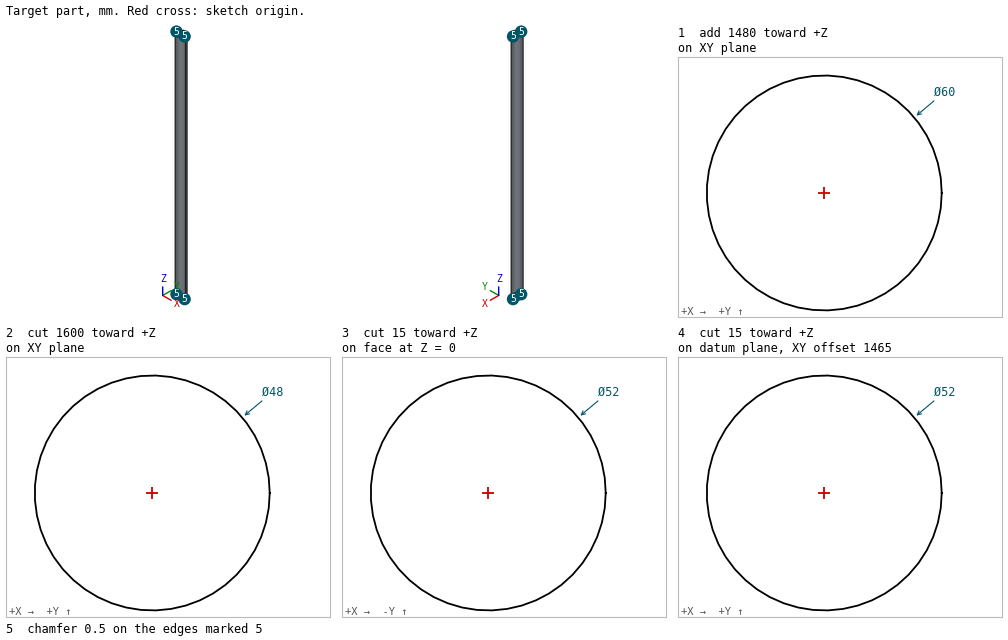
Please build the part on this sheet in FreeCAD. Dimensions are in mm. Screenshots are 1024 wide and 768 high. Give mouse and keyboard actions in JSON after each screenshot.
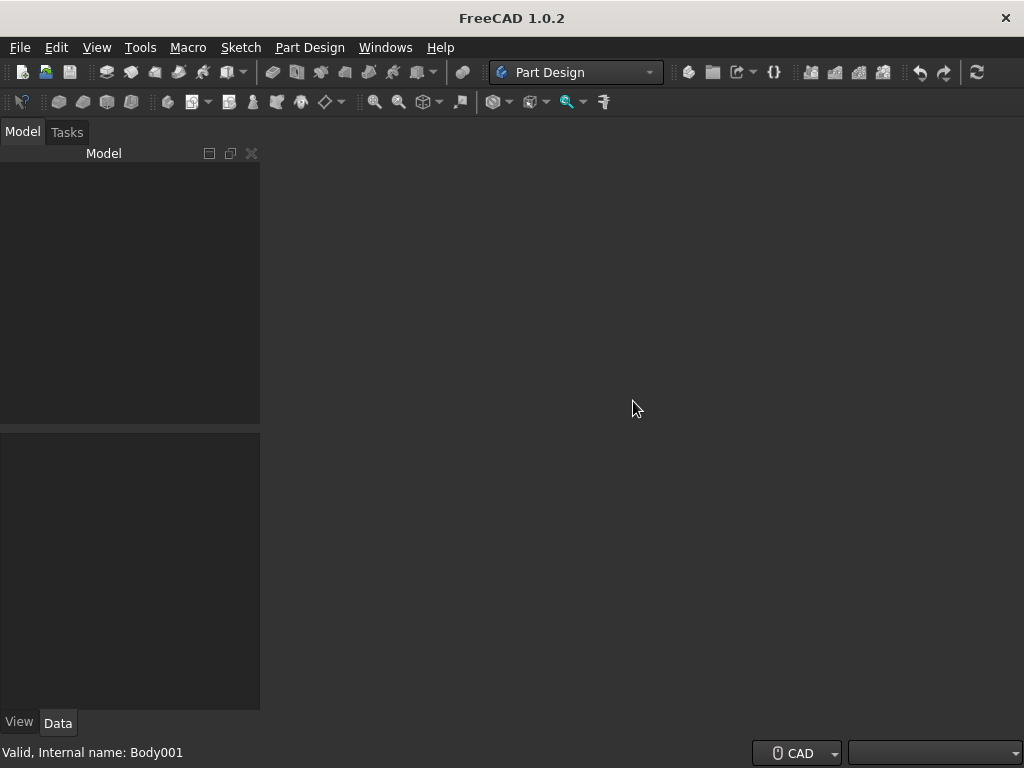
{"action": "left_click", "coordinate": [22, 72]}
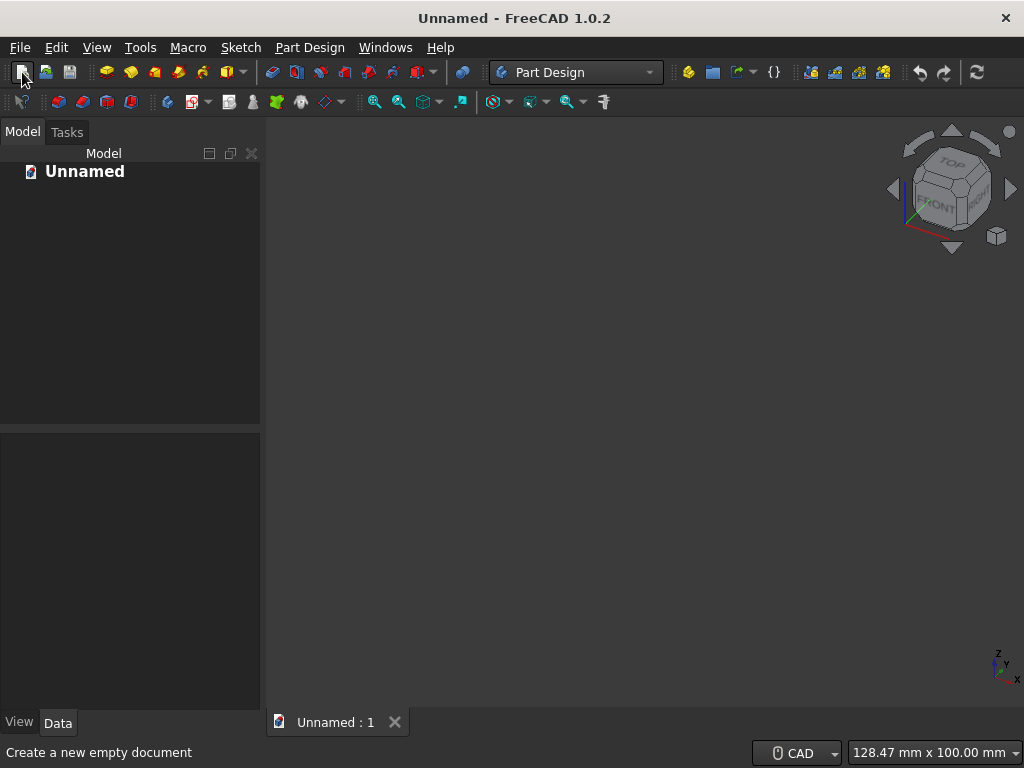
{"action": "left_click", "coordinate": [192, 102]}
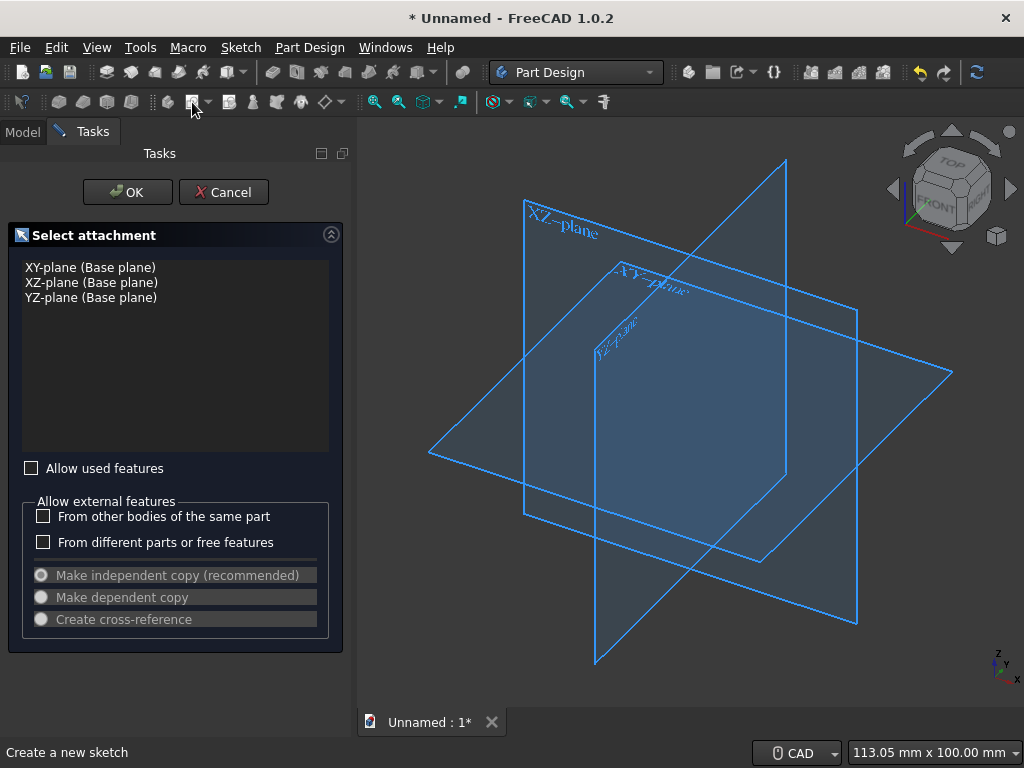
{"action": "left_click", "coordinate": [82, 268]}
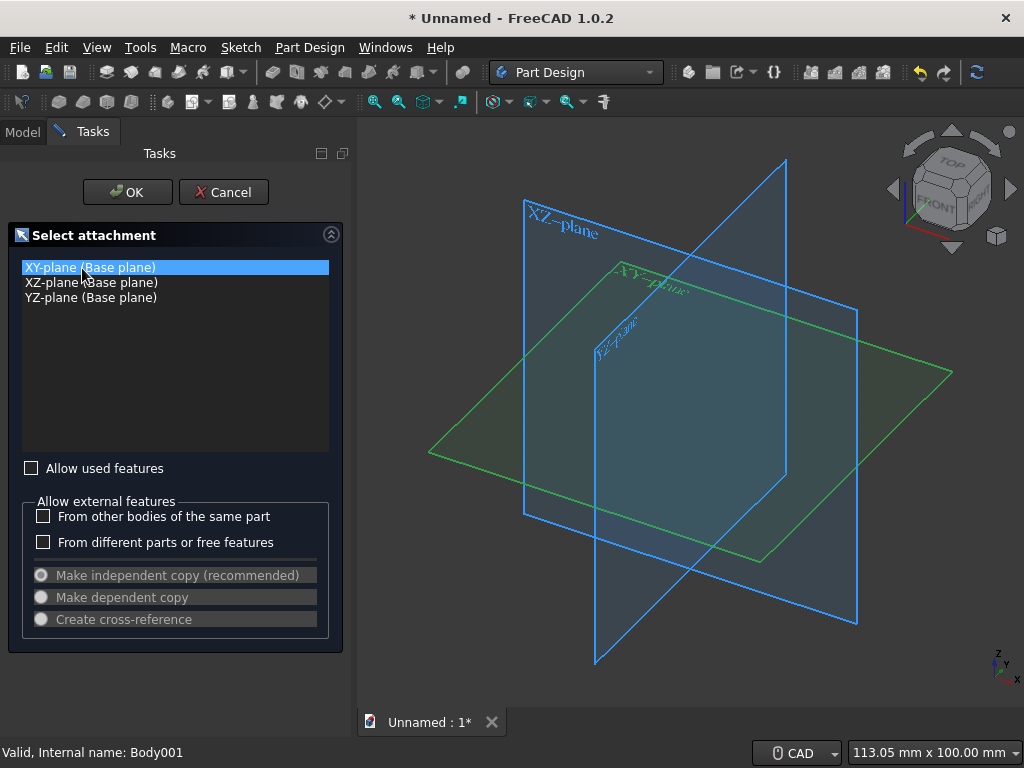
{"action": "left_click", "coordinate": [128, 192]}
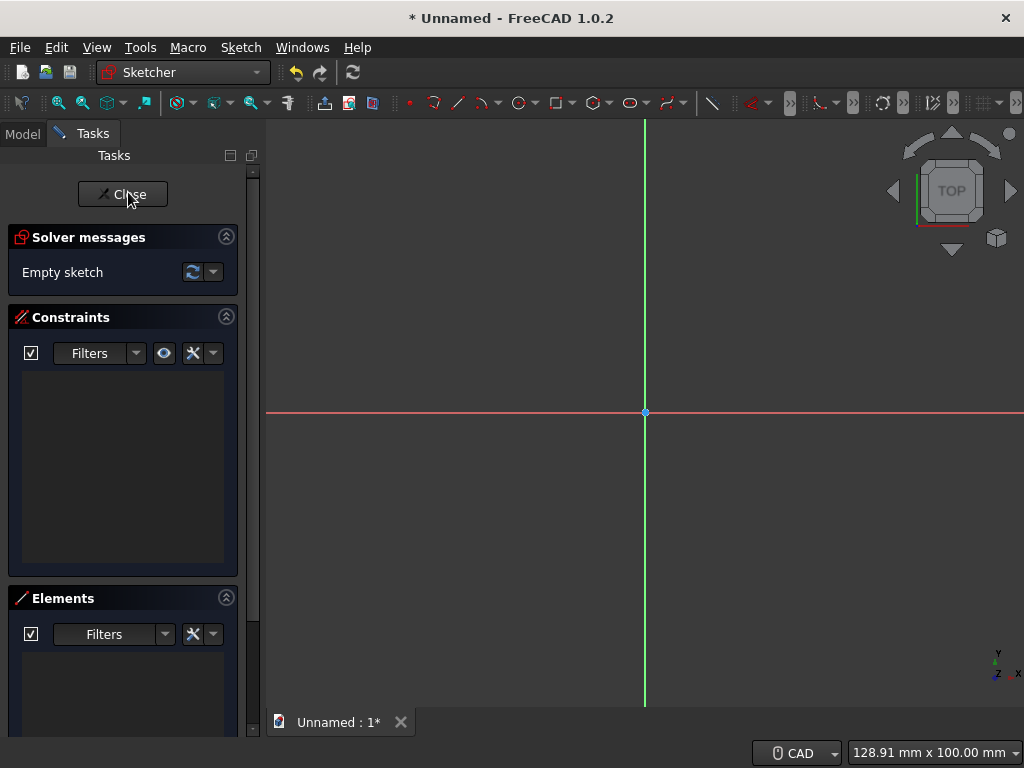
{"action": "left_click", "coordinate": [520, 104]}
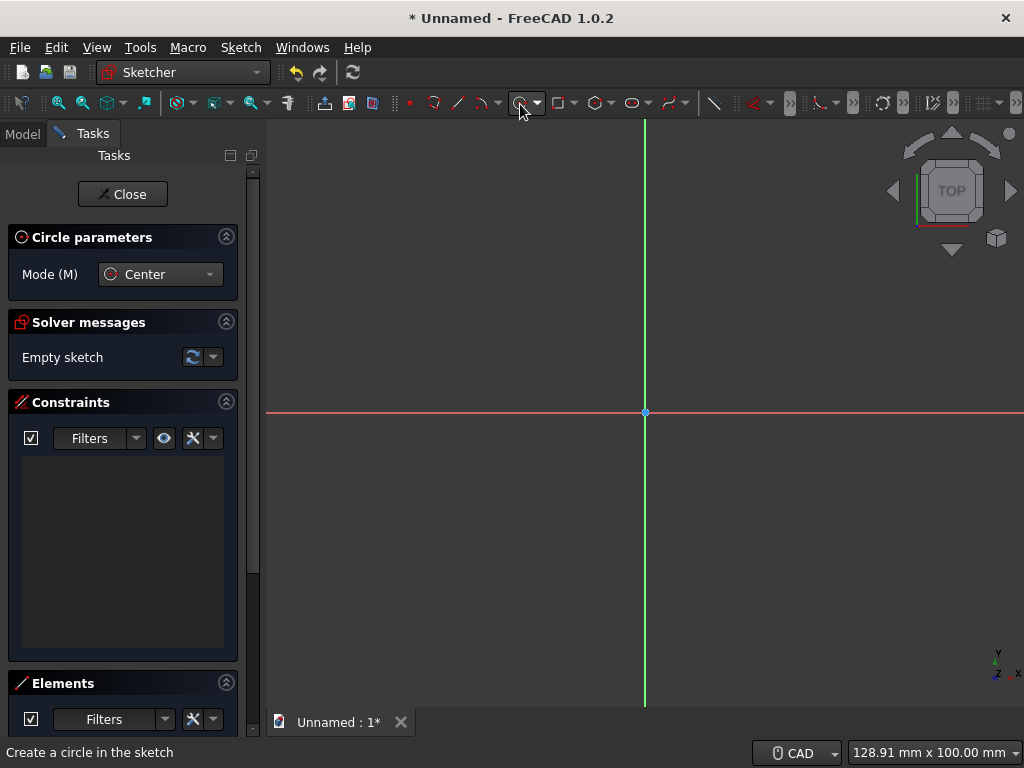
{"action": "left_click", "coordinate": [645, 413]}
{"action": "mouse_move", "coordinate": [770, 288]}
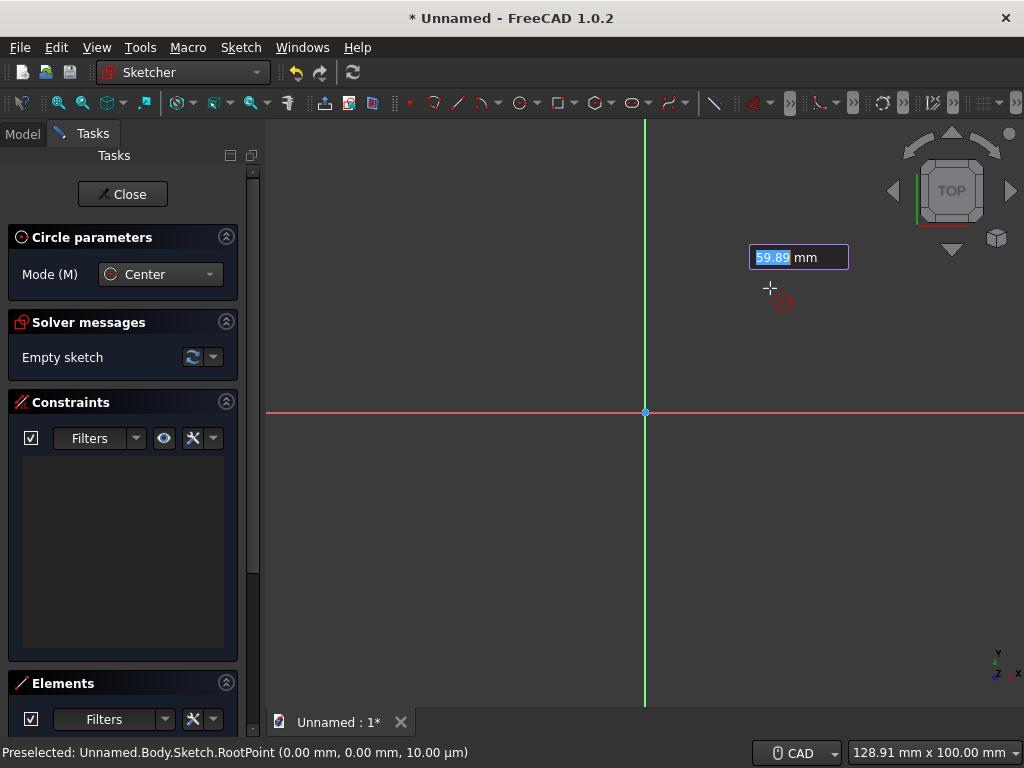
{"action": "type", "text": "60"}
{"action": "key", "text": "Return"}
{"action": "key", "text": "Escape"}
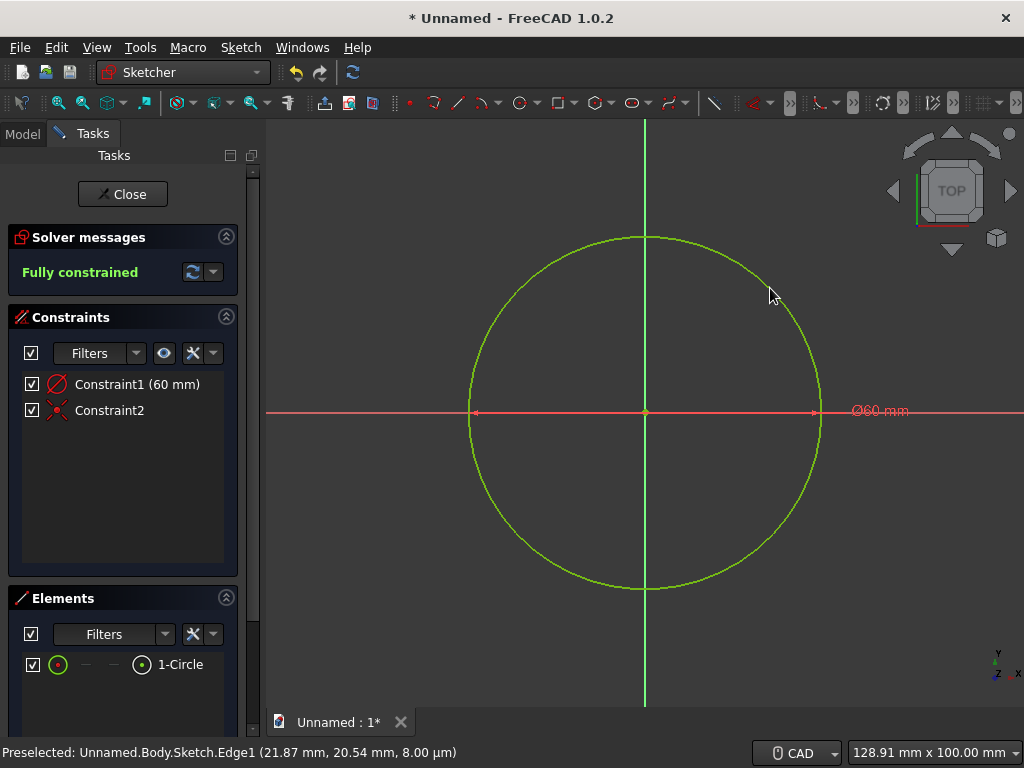
{"action": "left_click", "coordinate": [123, 194]}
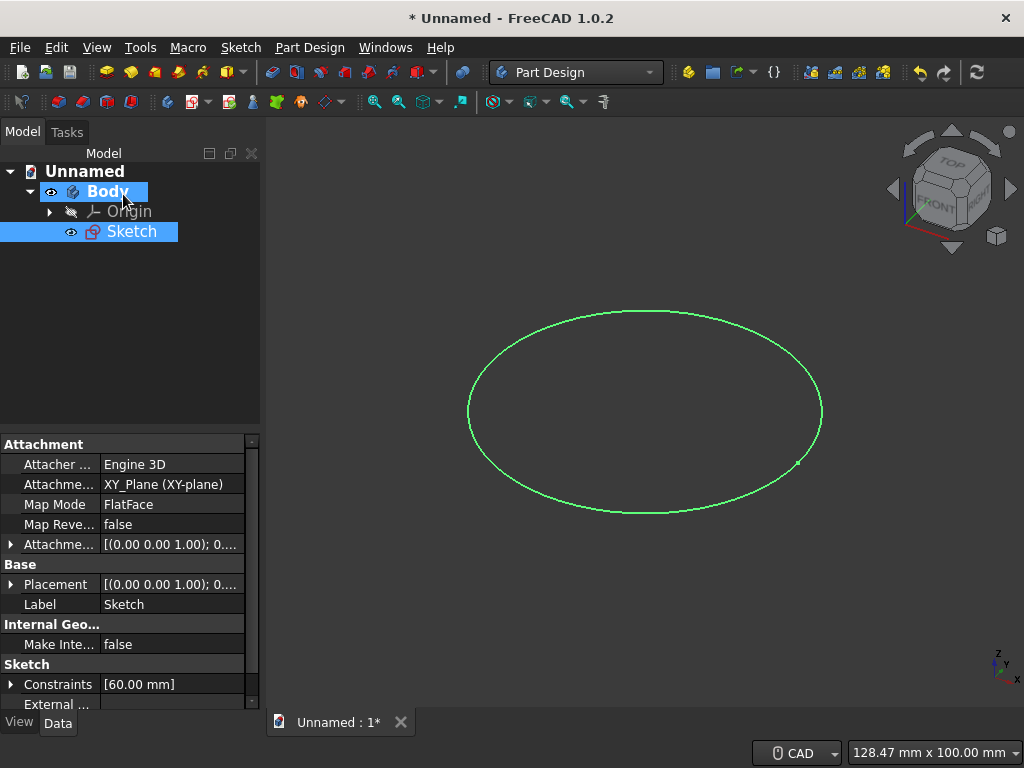
{"action": "left_click", "coordinate": [108, 72]}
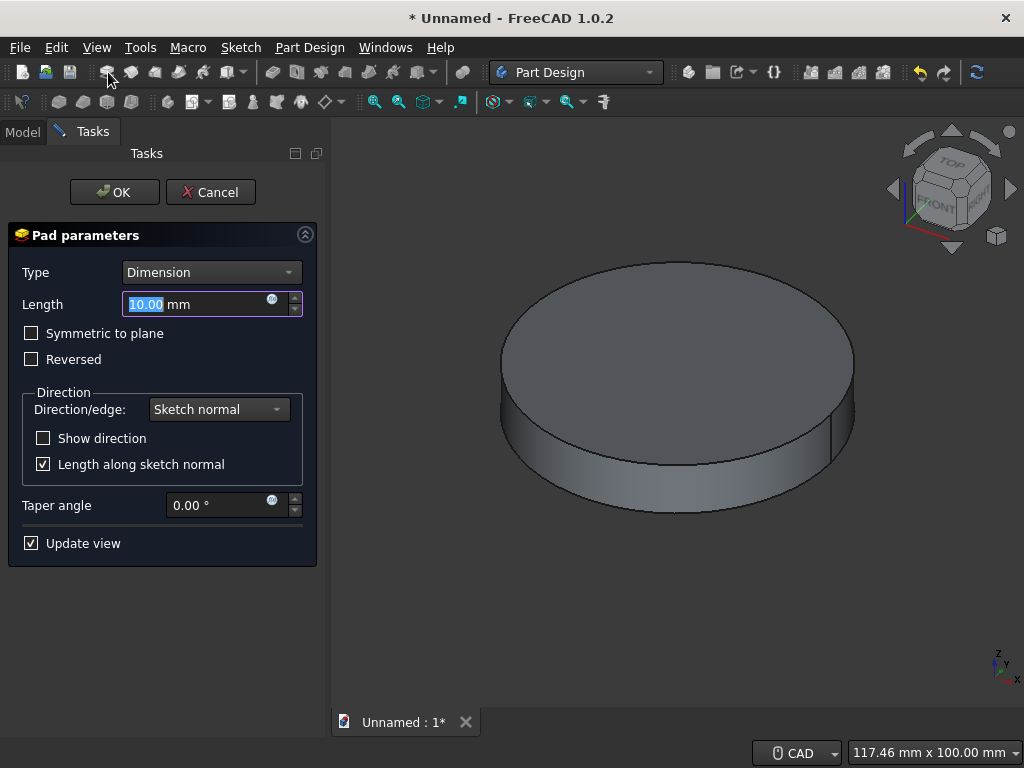
{"action": "type", "text": "1480"}
{"action": "key", "text": "Tab"}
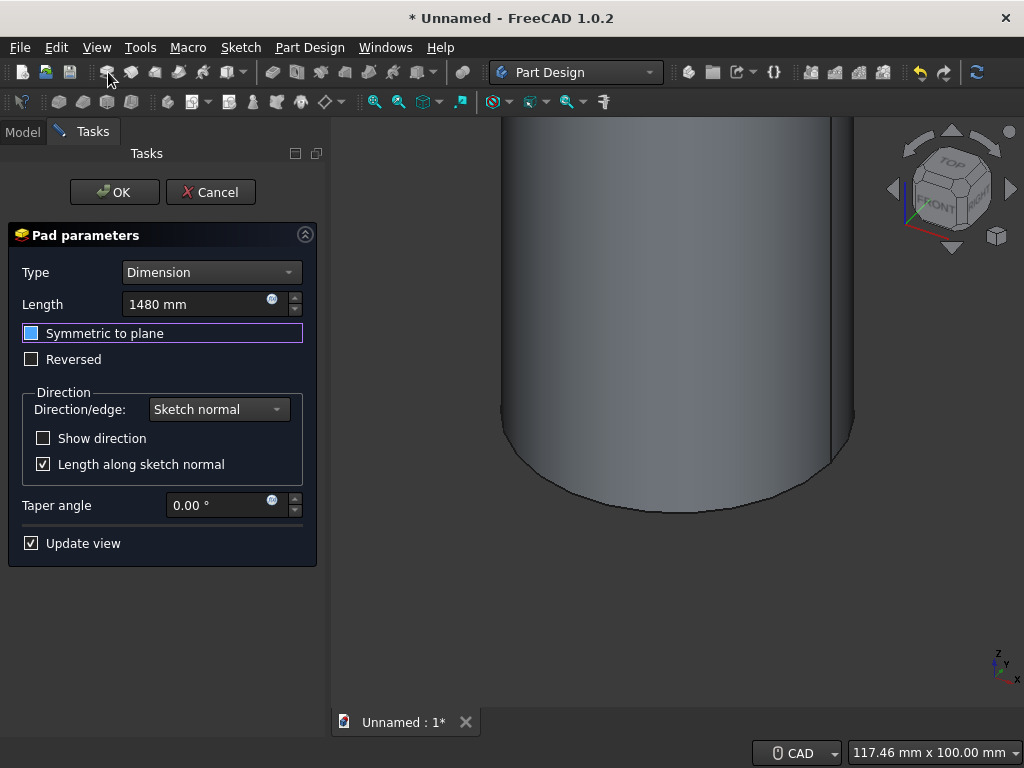
{"action": "left_click", "coordinate": [115, 192]}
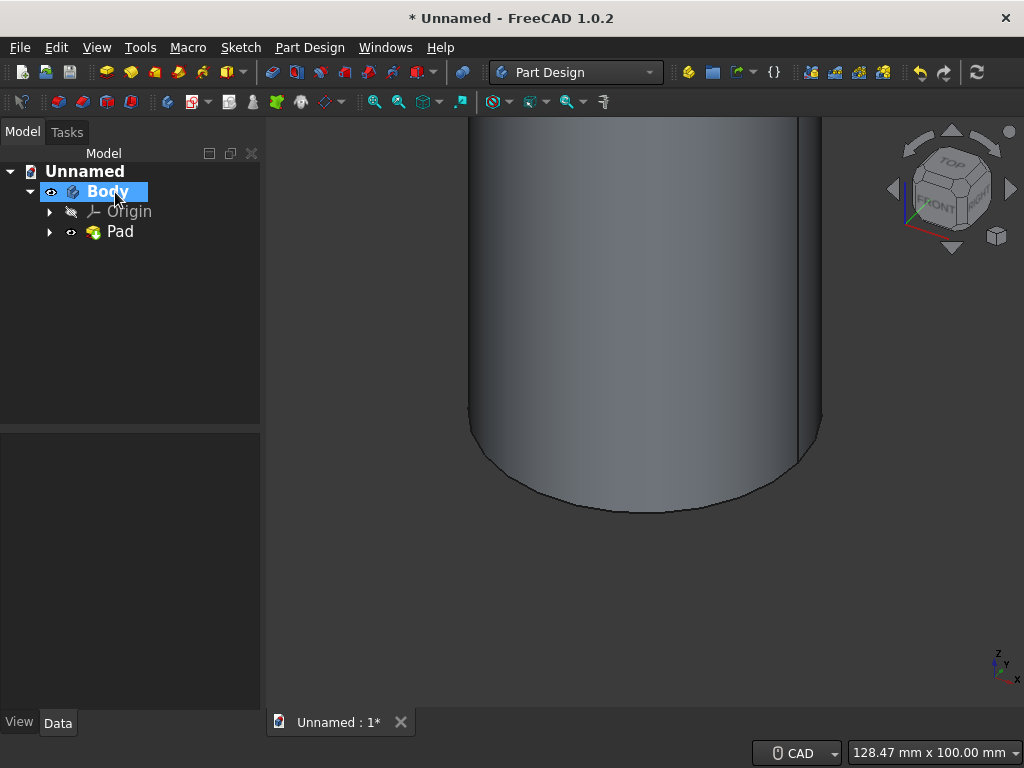
{"action": "left_click", "coordinate": [376, 102]}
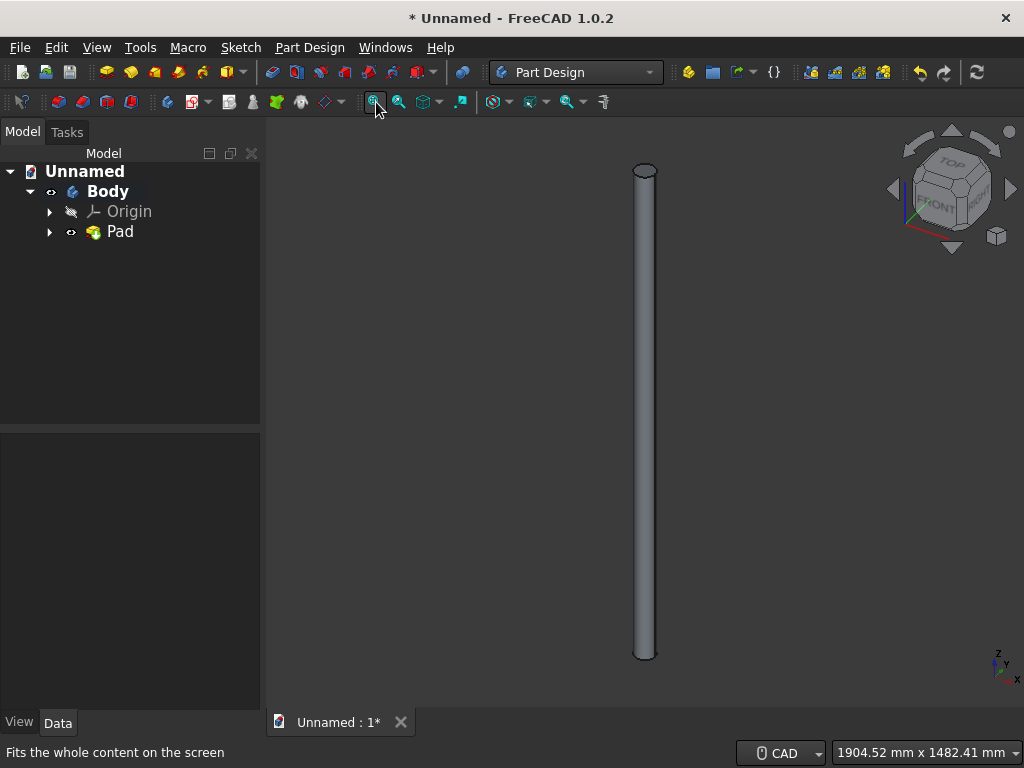
{"action": "left_click", "coordinate": [192, 102]}